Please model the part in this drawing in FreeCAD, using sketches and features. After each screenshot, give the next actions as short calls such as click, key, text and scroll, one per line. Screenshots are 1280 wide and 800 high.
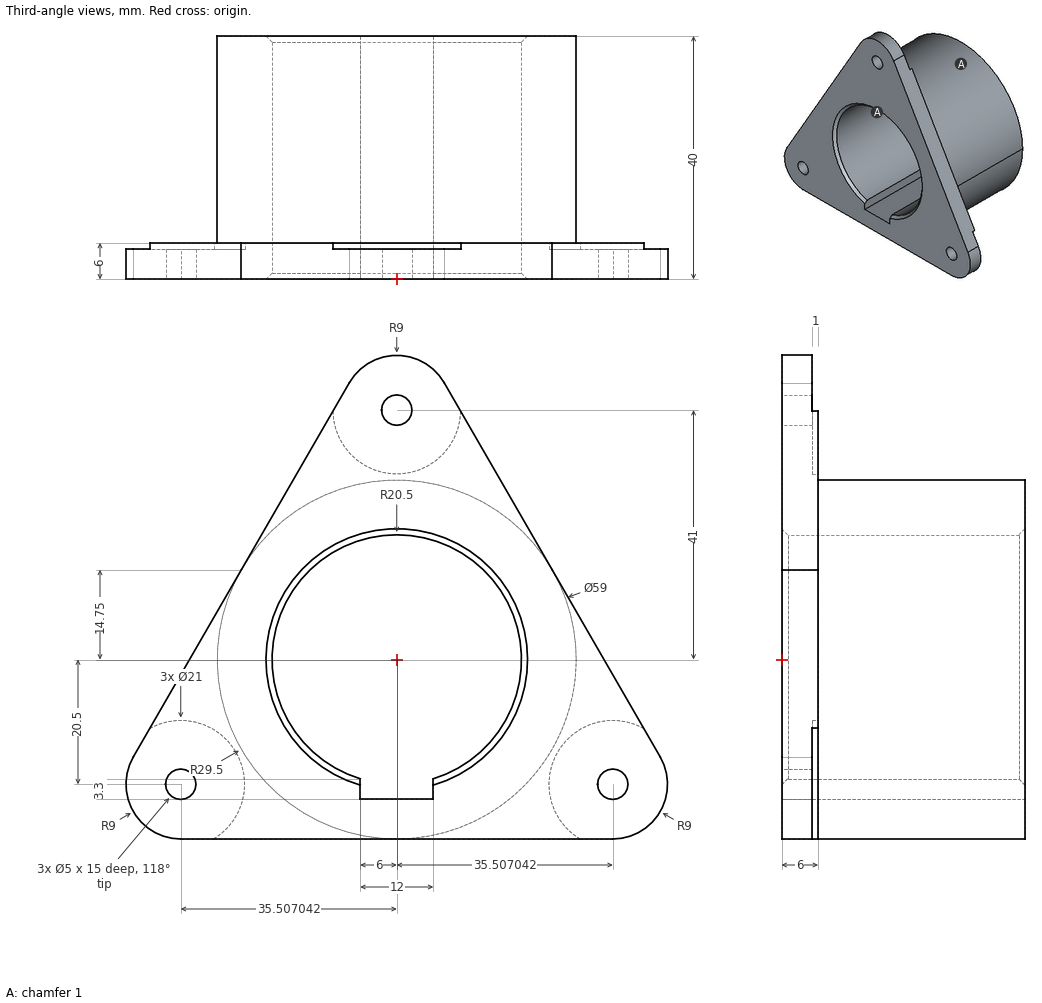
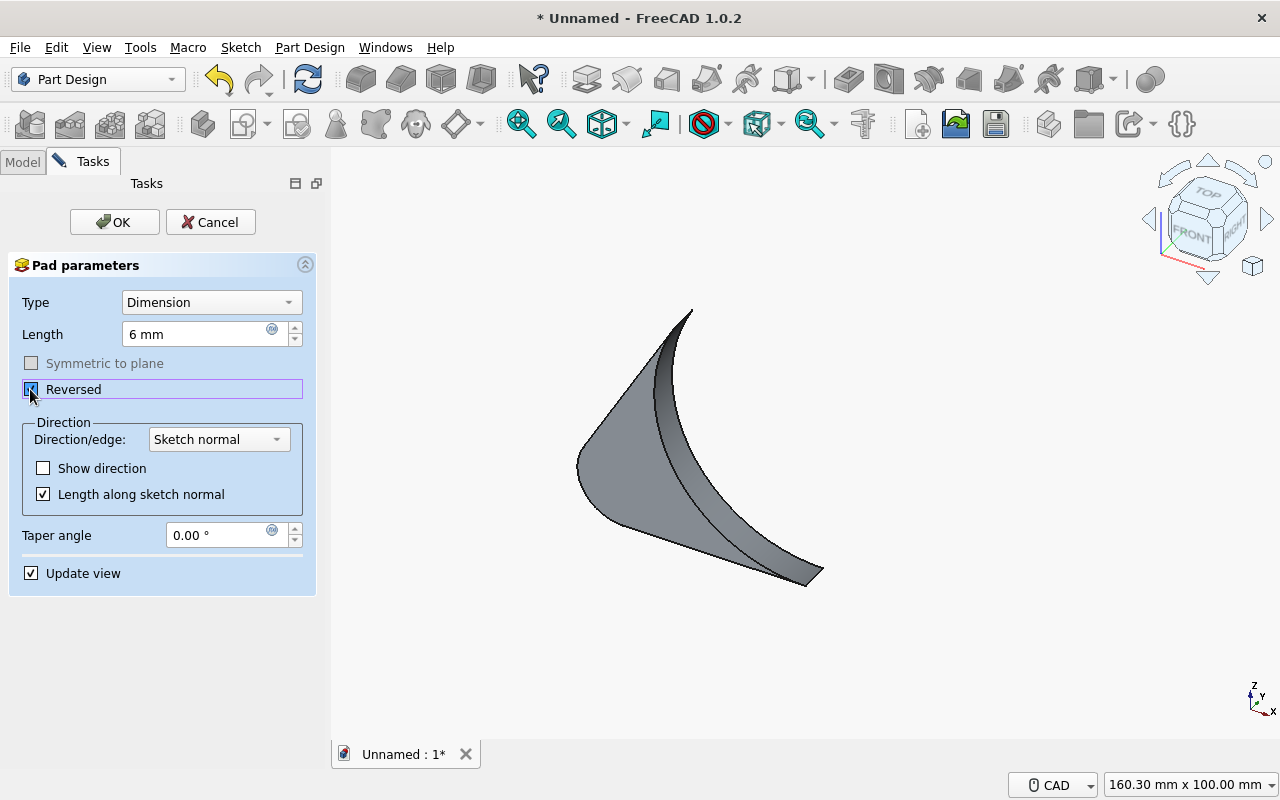
click(115, 222)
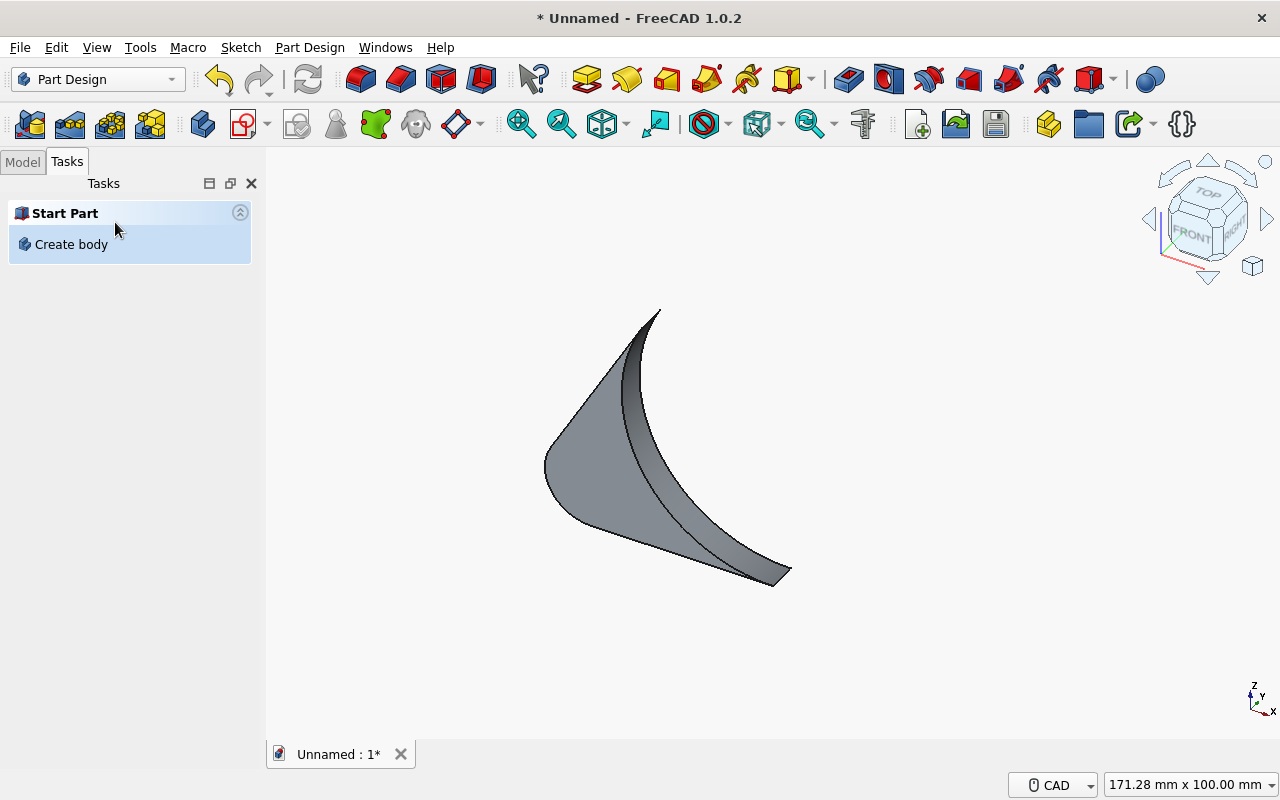
click(204, 124)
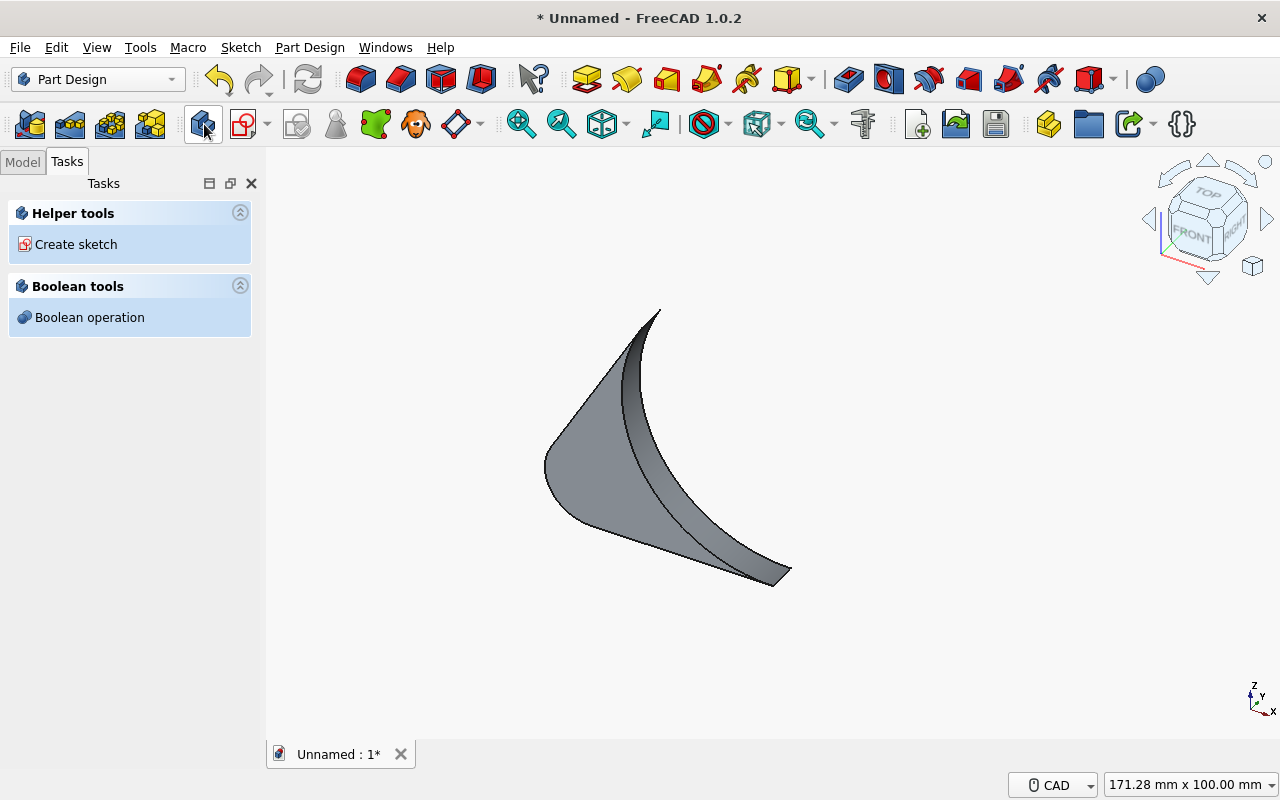
click(306, 699)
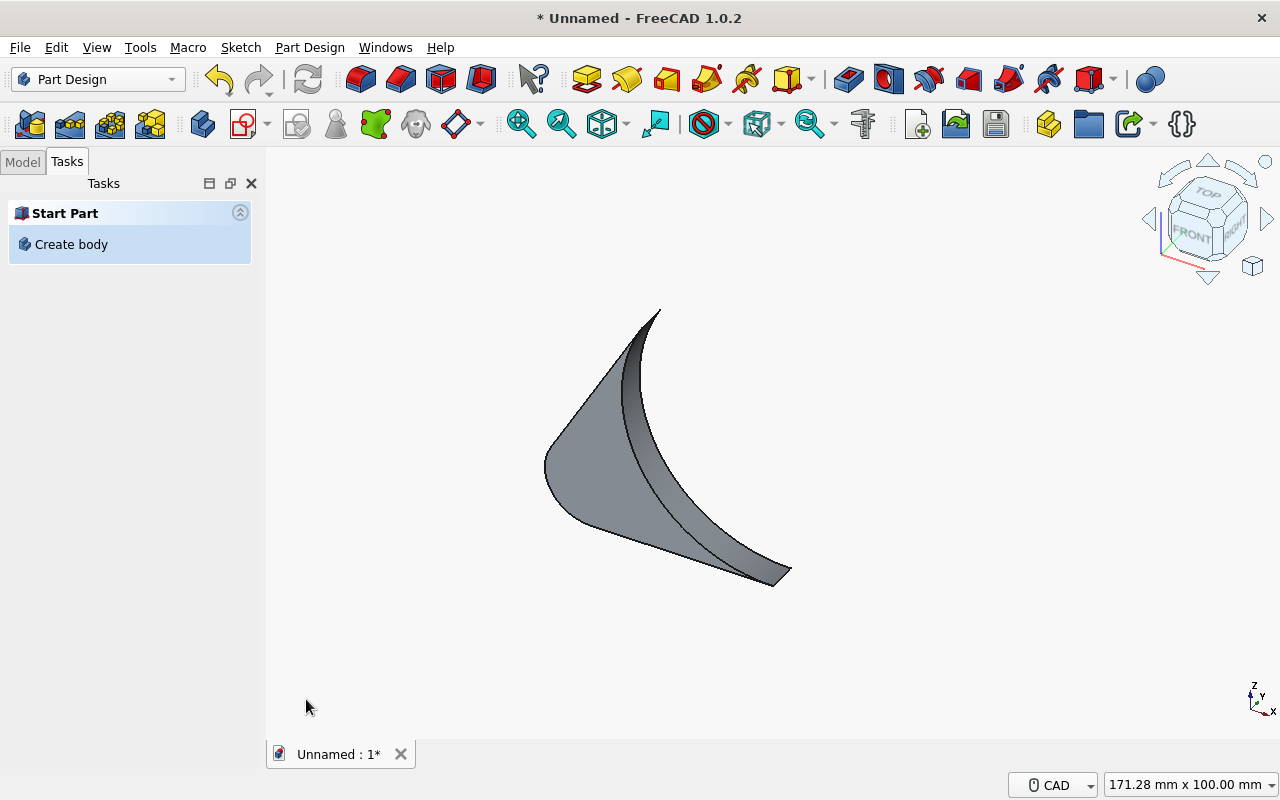
click(244, 124)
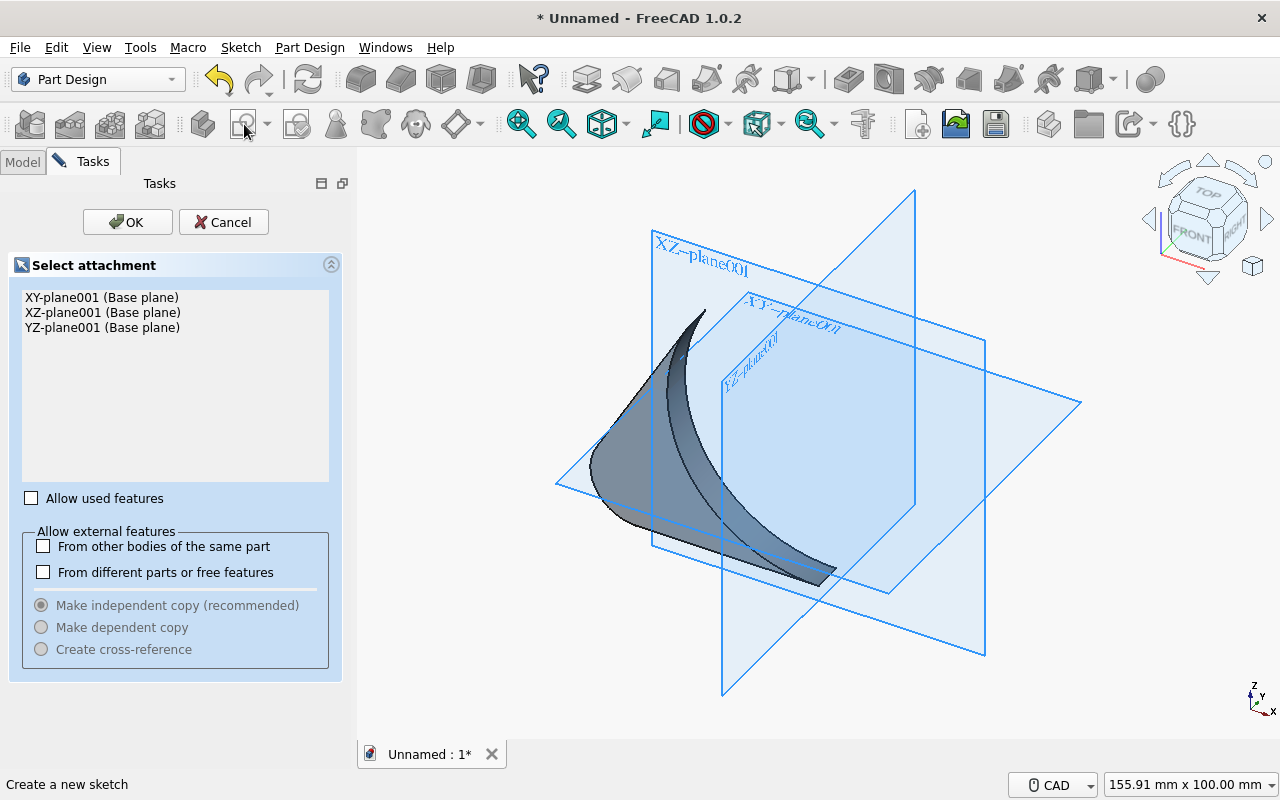
click(82, 312)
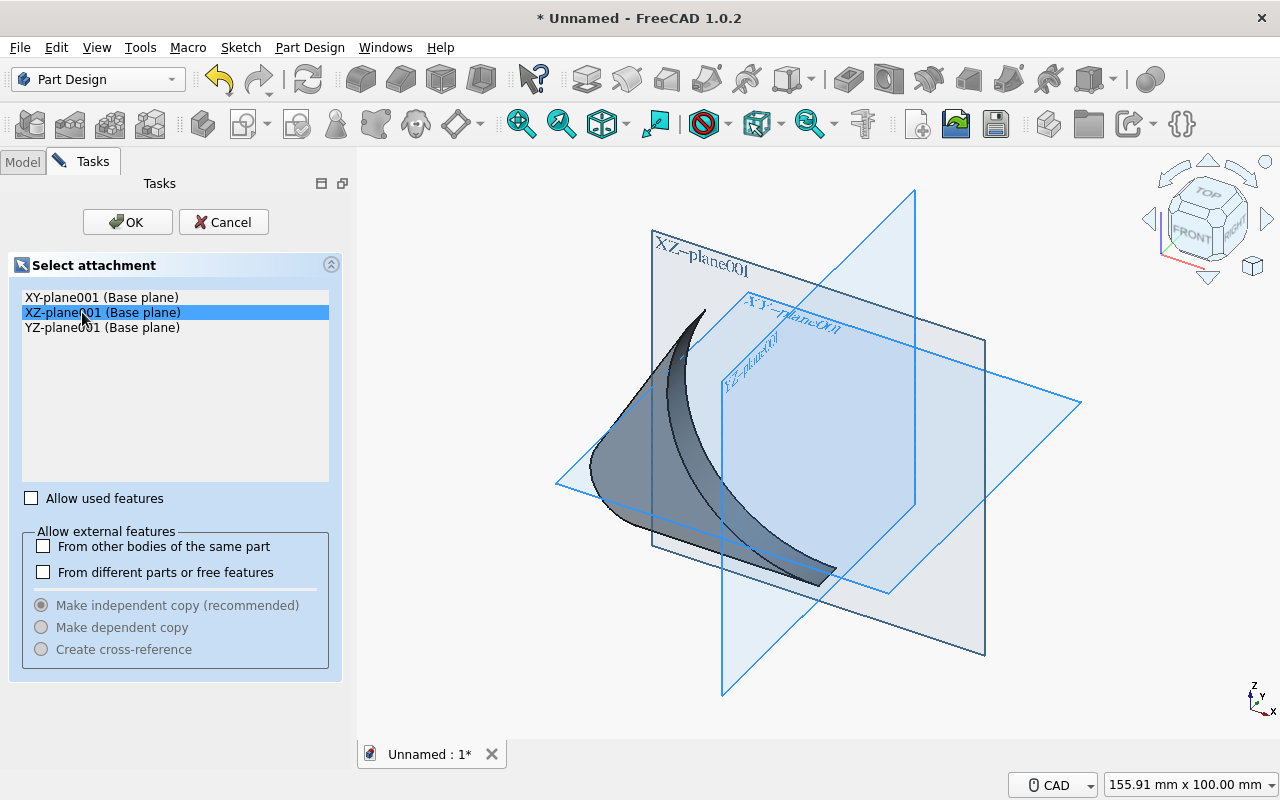
click(128, 222)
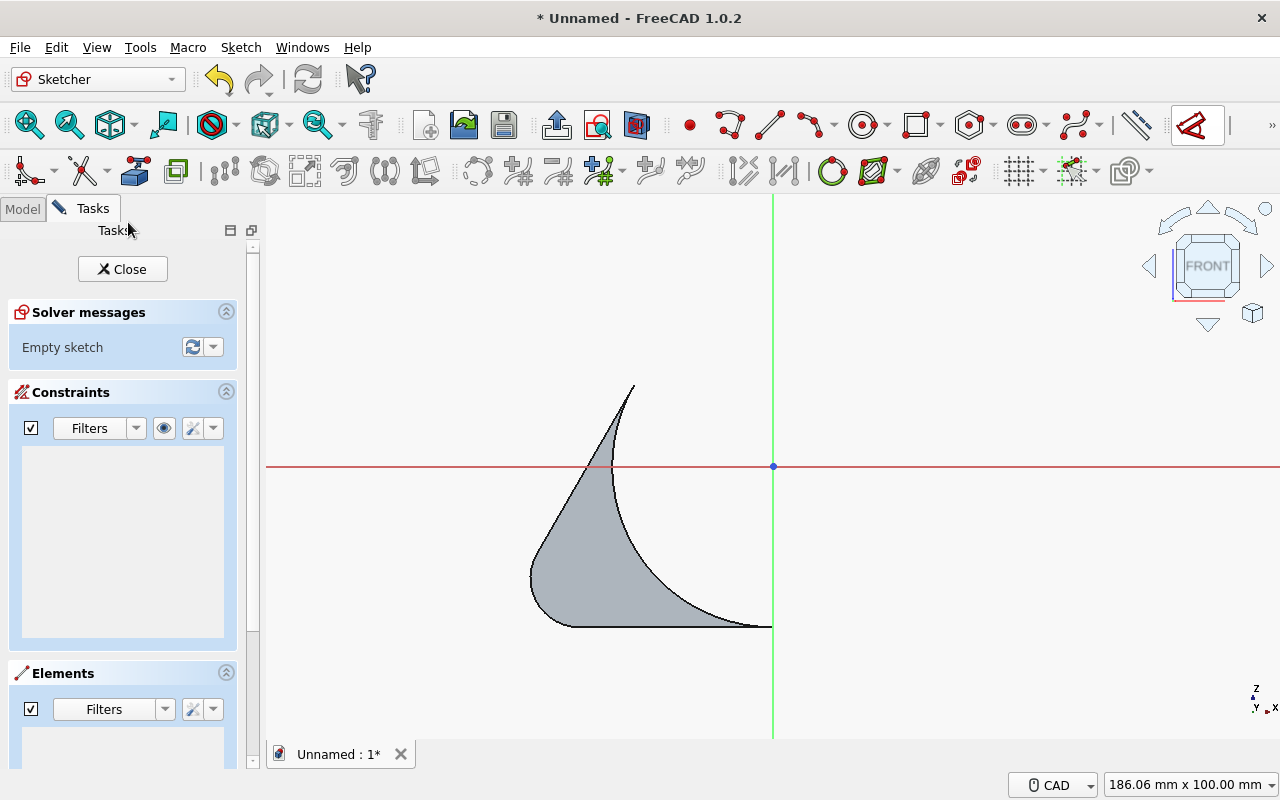
scroll(395, 711, down, 1)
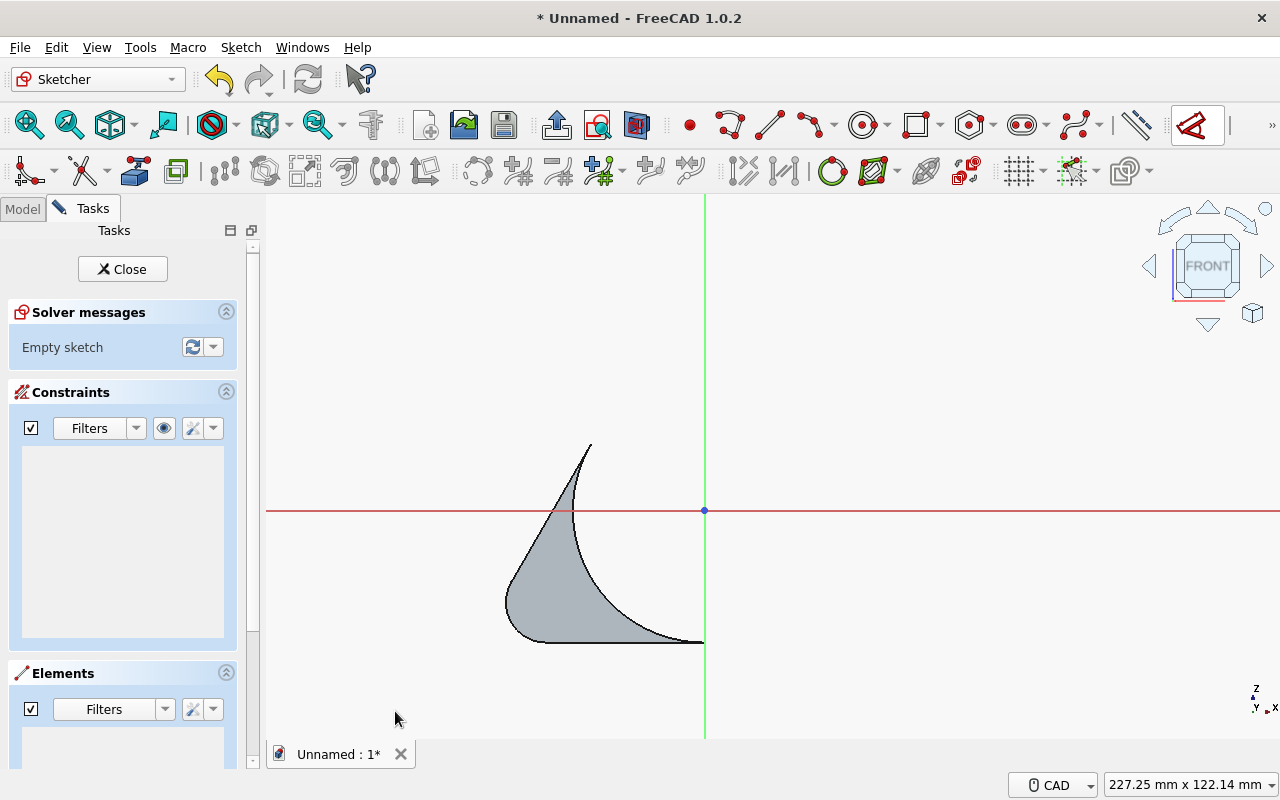
scroll(705, 263, up, 2)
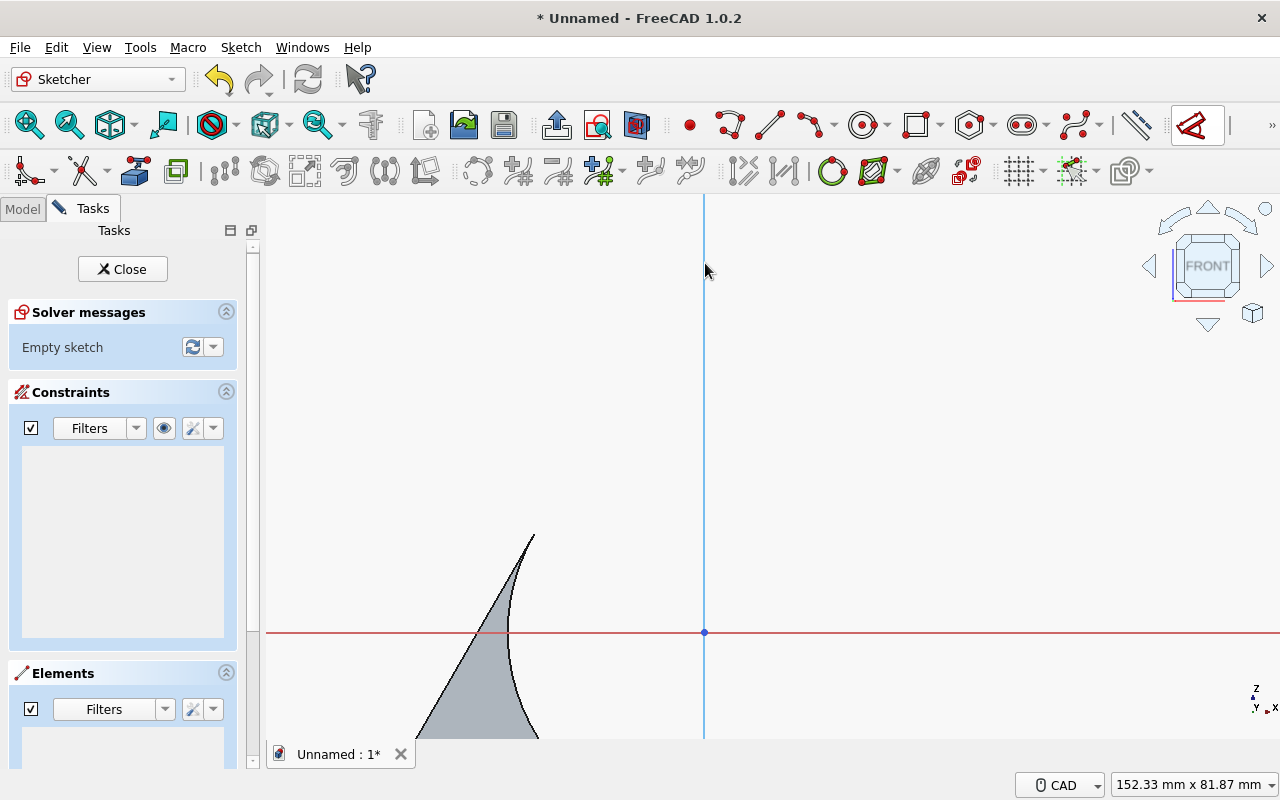
click(770, 126)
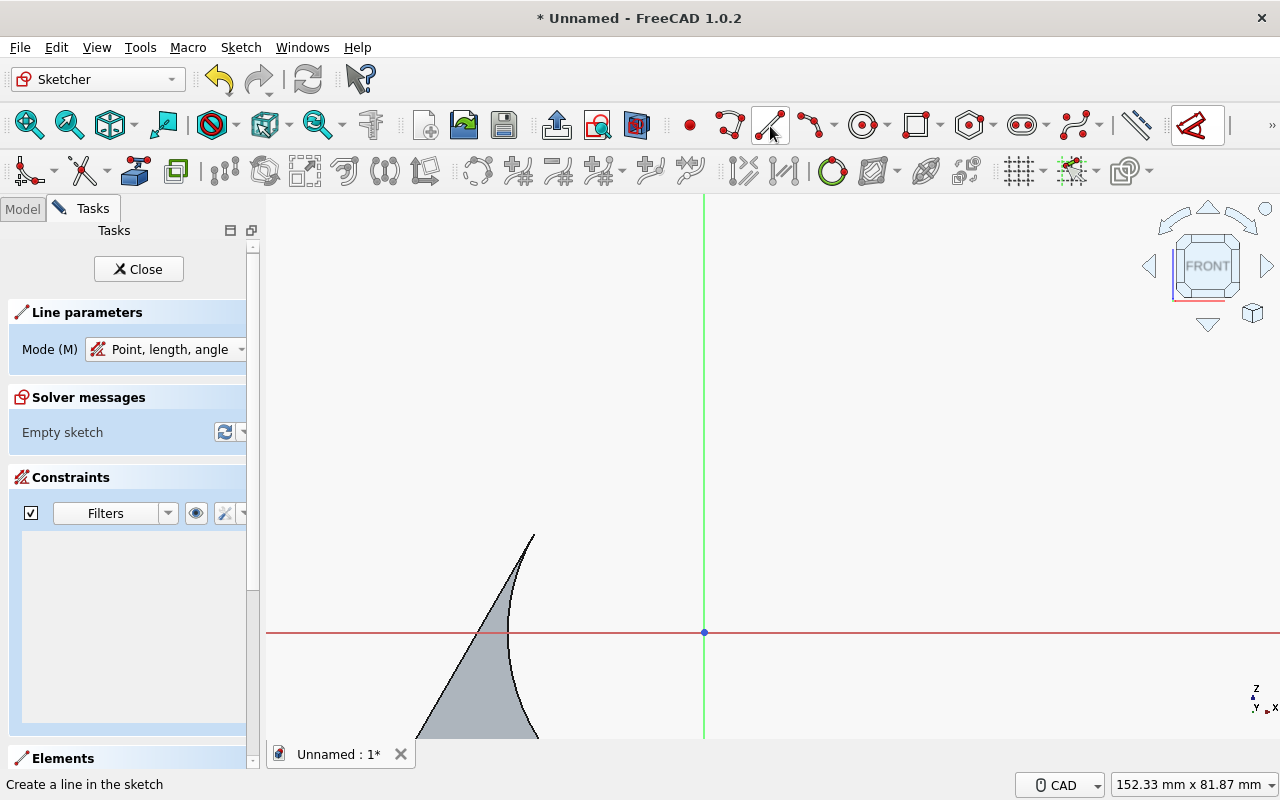
click(534, 535)
click(652, 330)